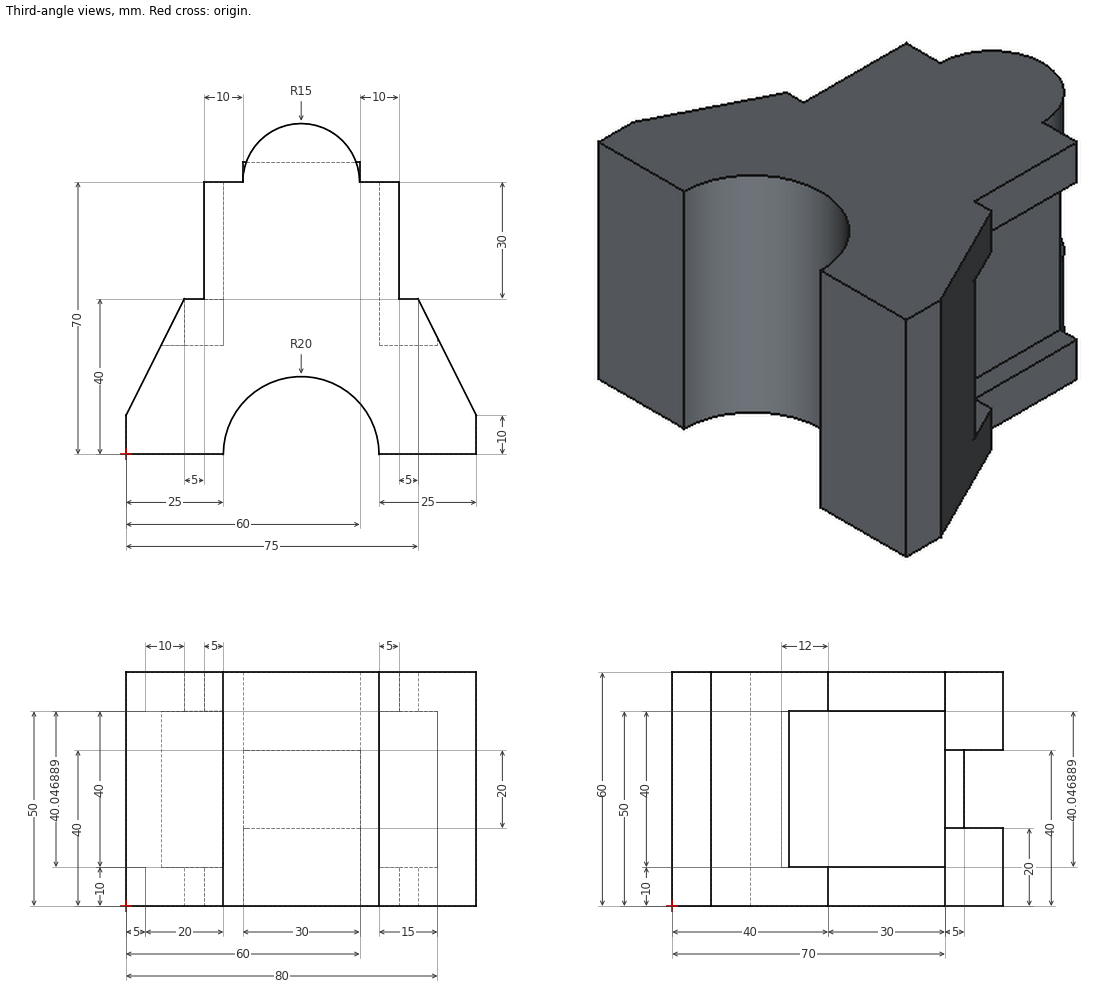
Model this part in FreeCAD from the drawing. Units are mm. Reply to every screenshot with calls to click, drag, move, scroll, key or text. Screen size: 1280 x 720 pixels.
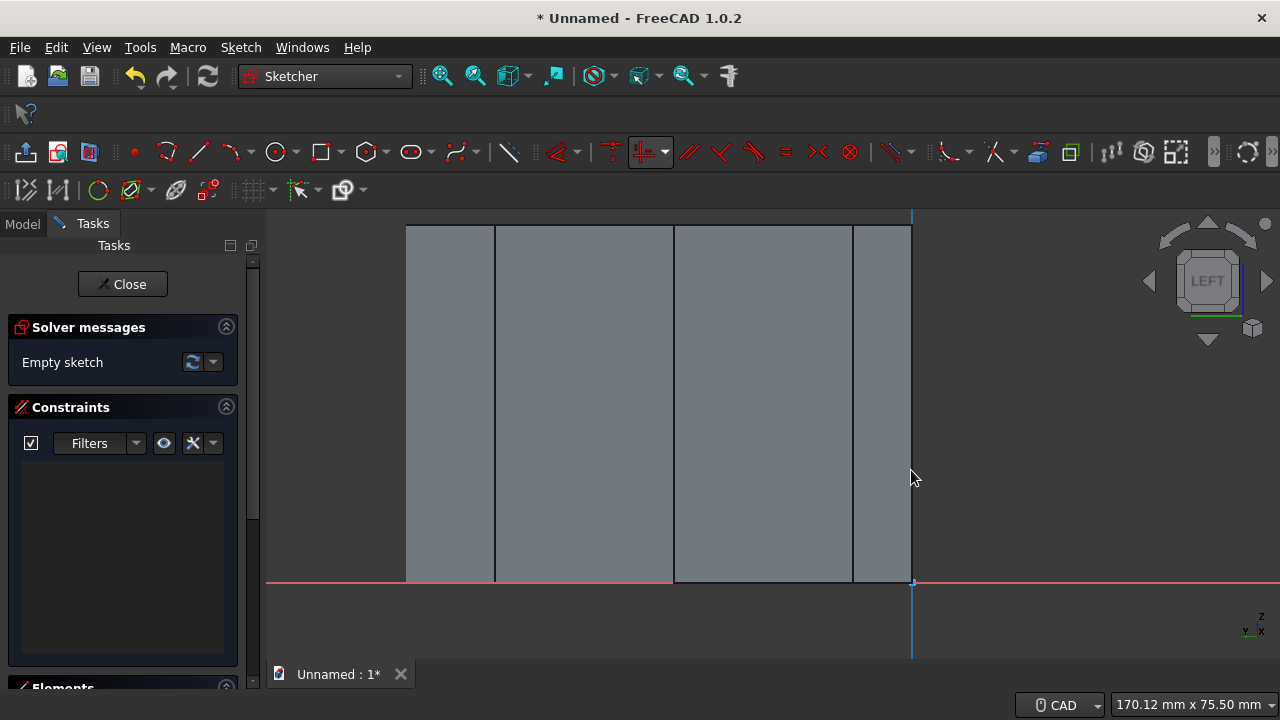
key(g)
key(r)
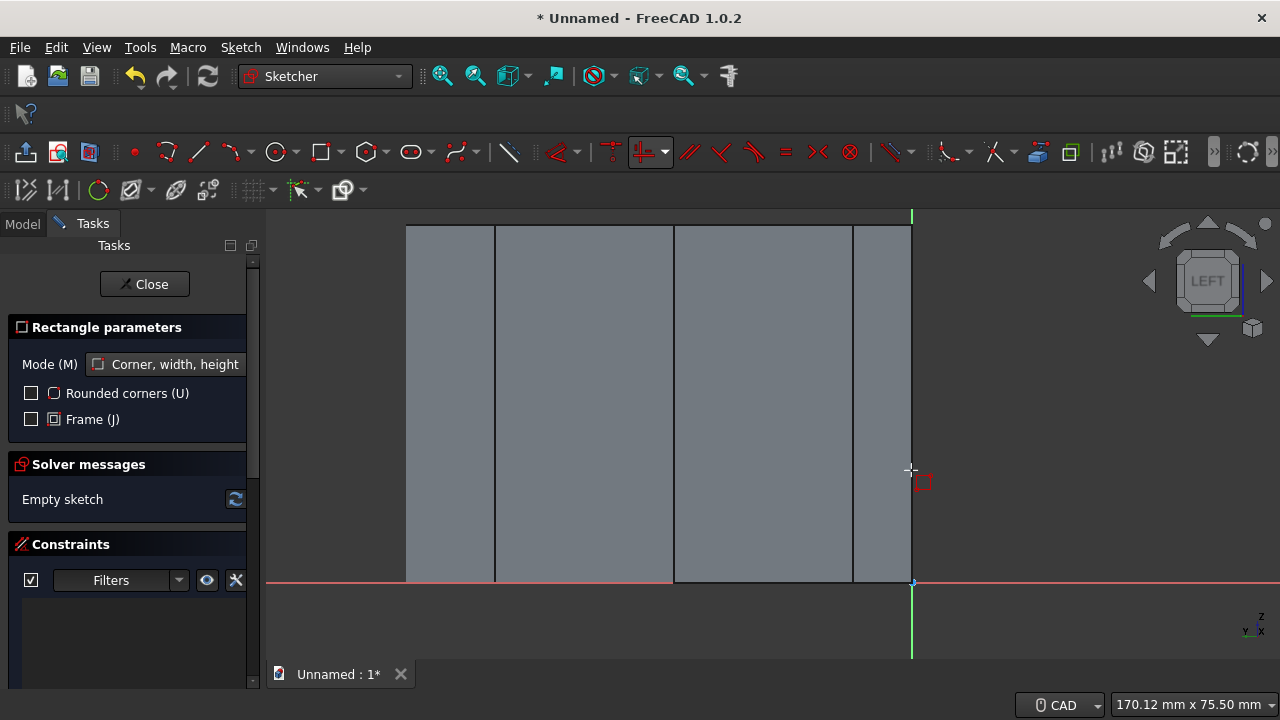
click(495, 284)
click(674, 523)
key(Escape)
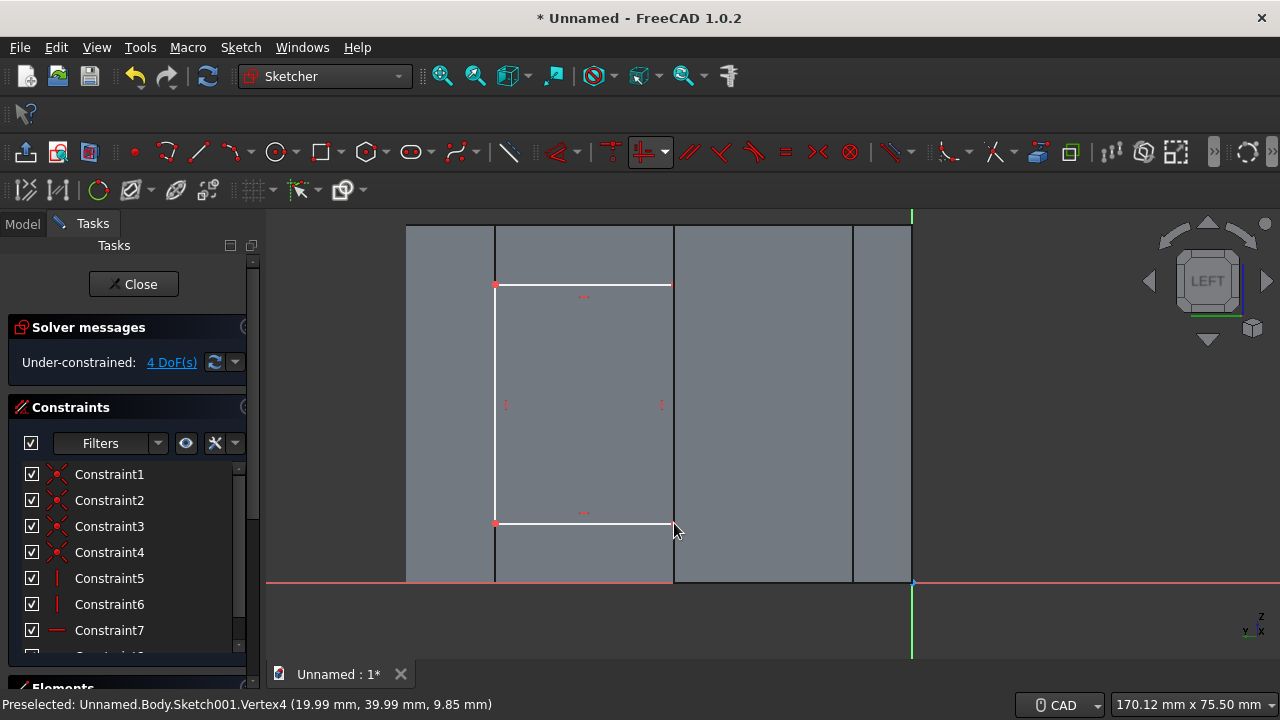
key(d)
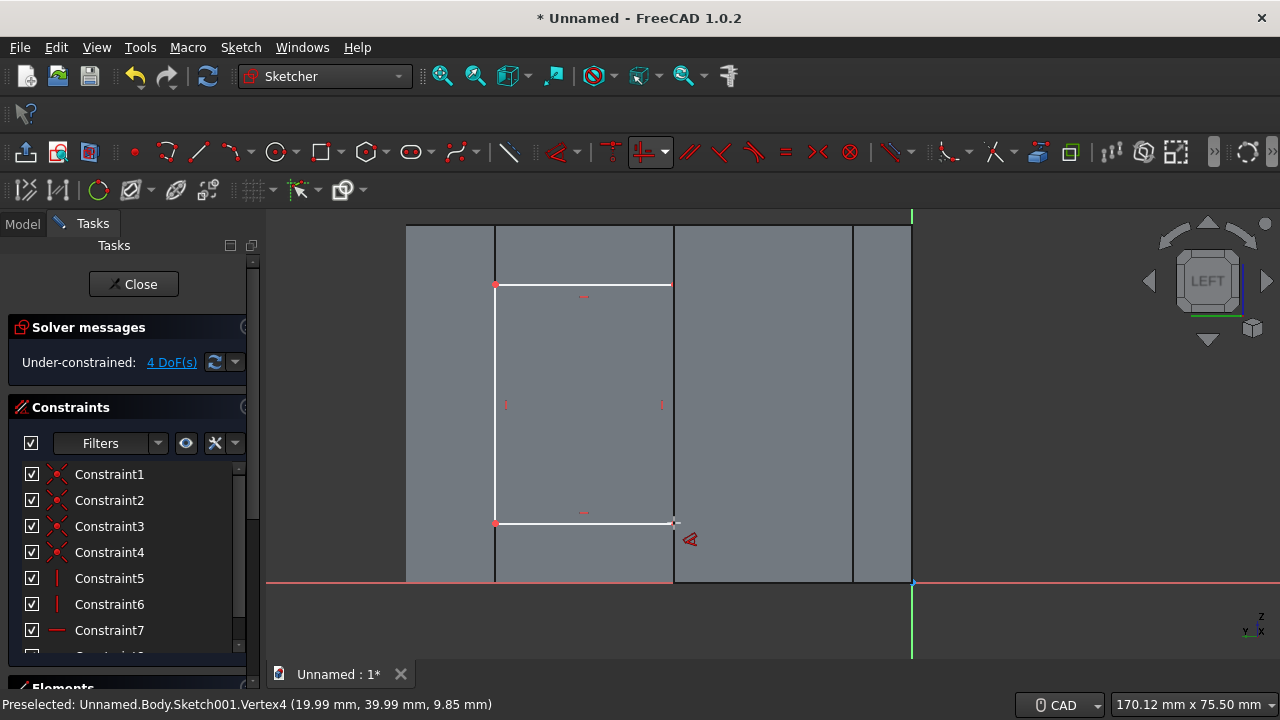
click(549, 524)
click(584, 558)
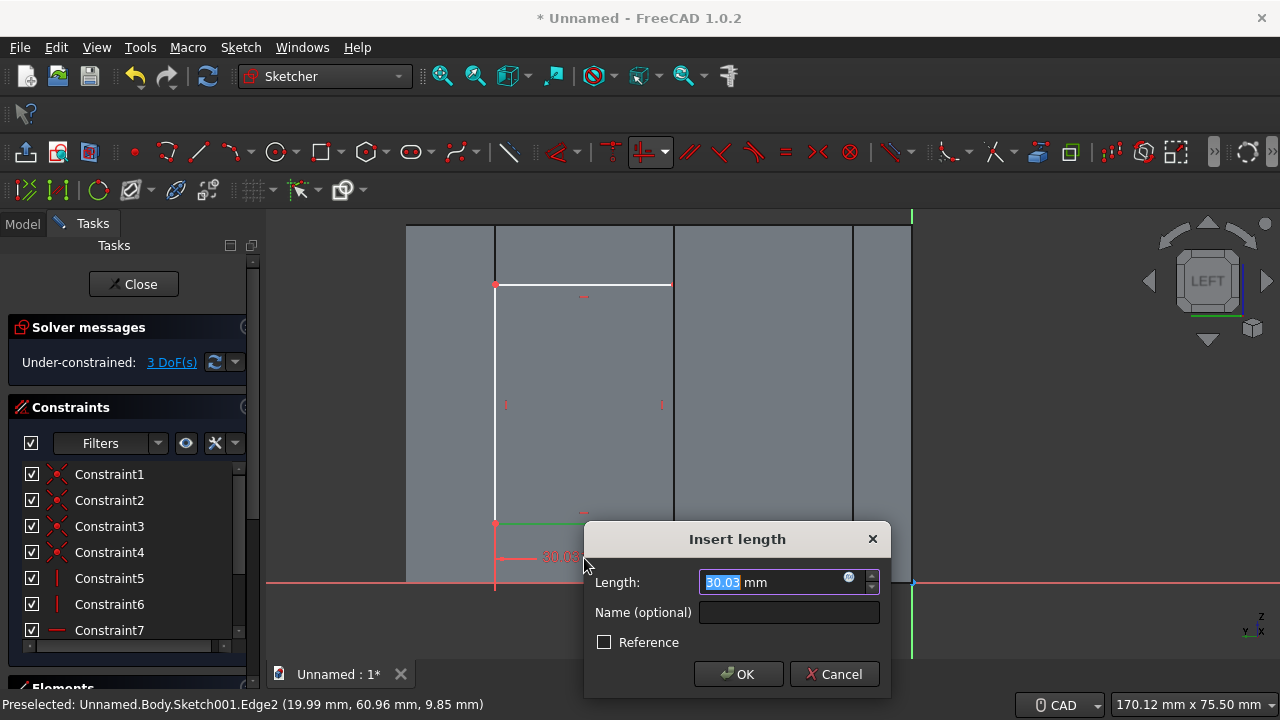
text(30)
key(Return)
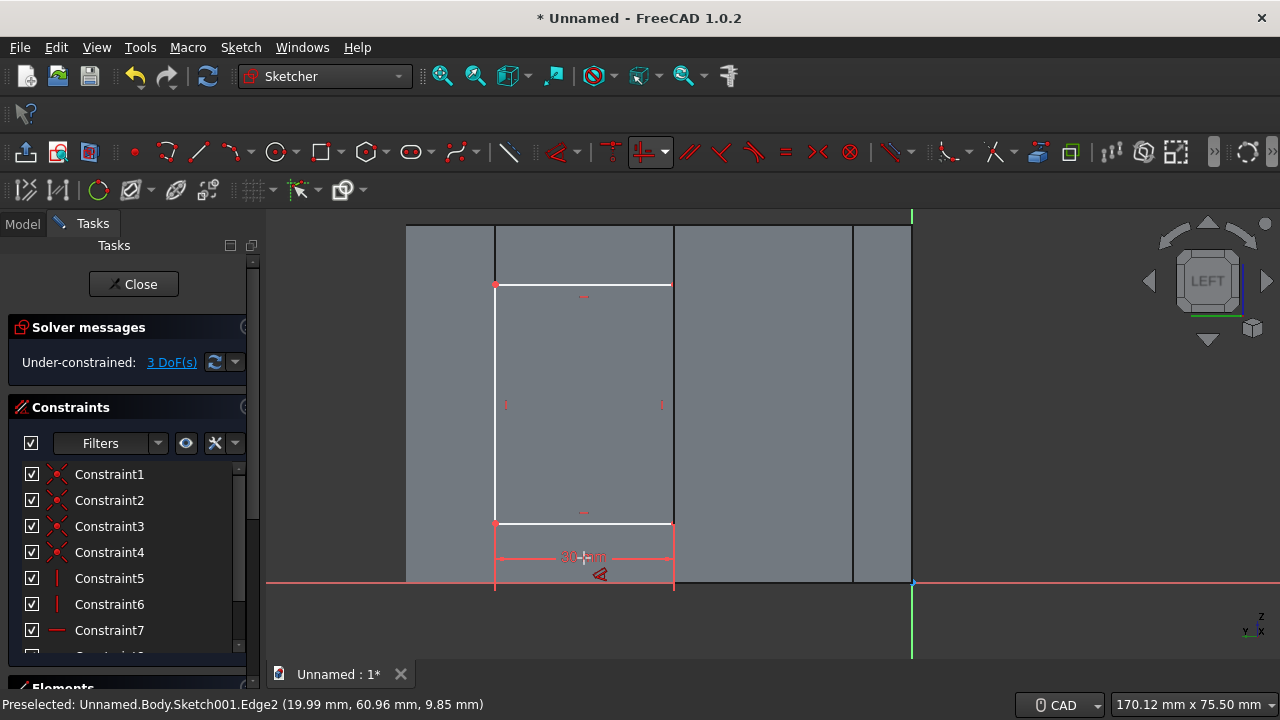
click(495, 285)
click(704, 617)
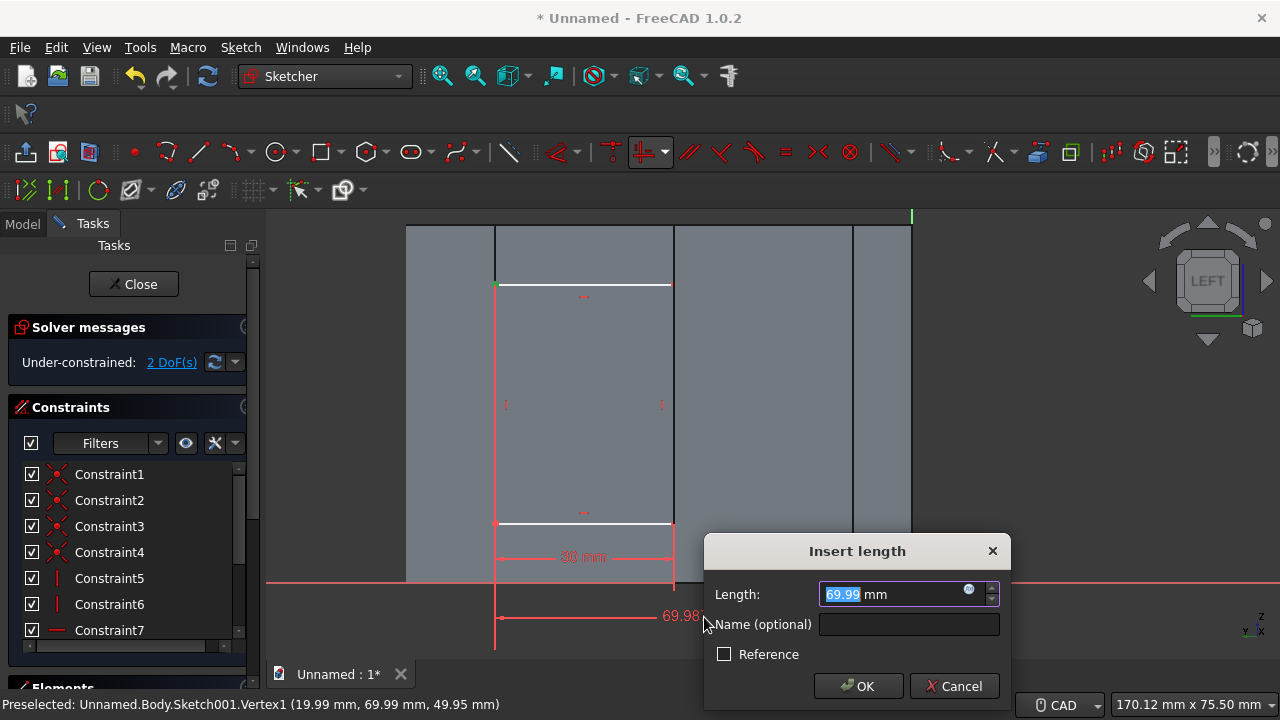
text(70)
key(Return)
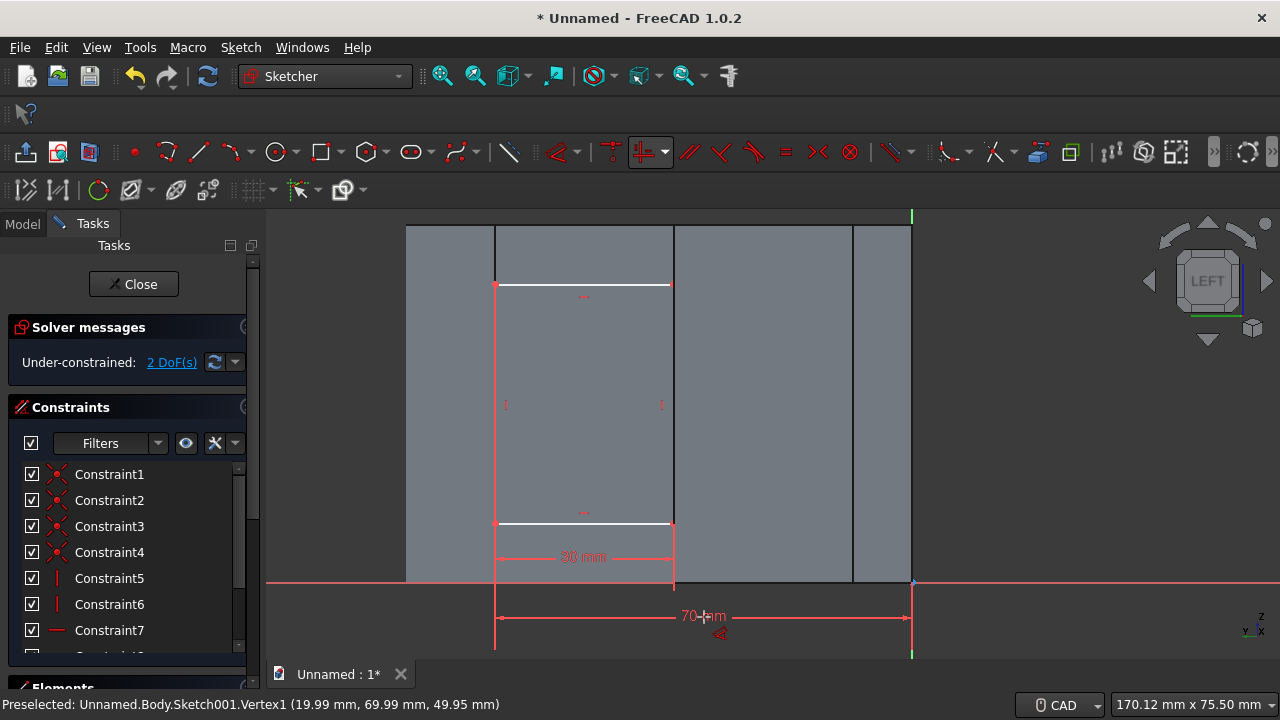
click(495, 524)
click(946, 553)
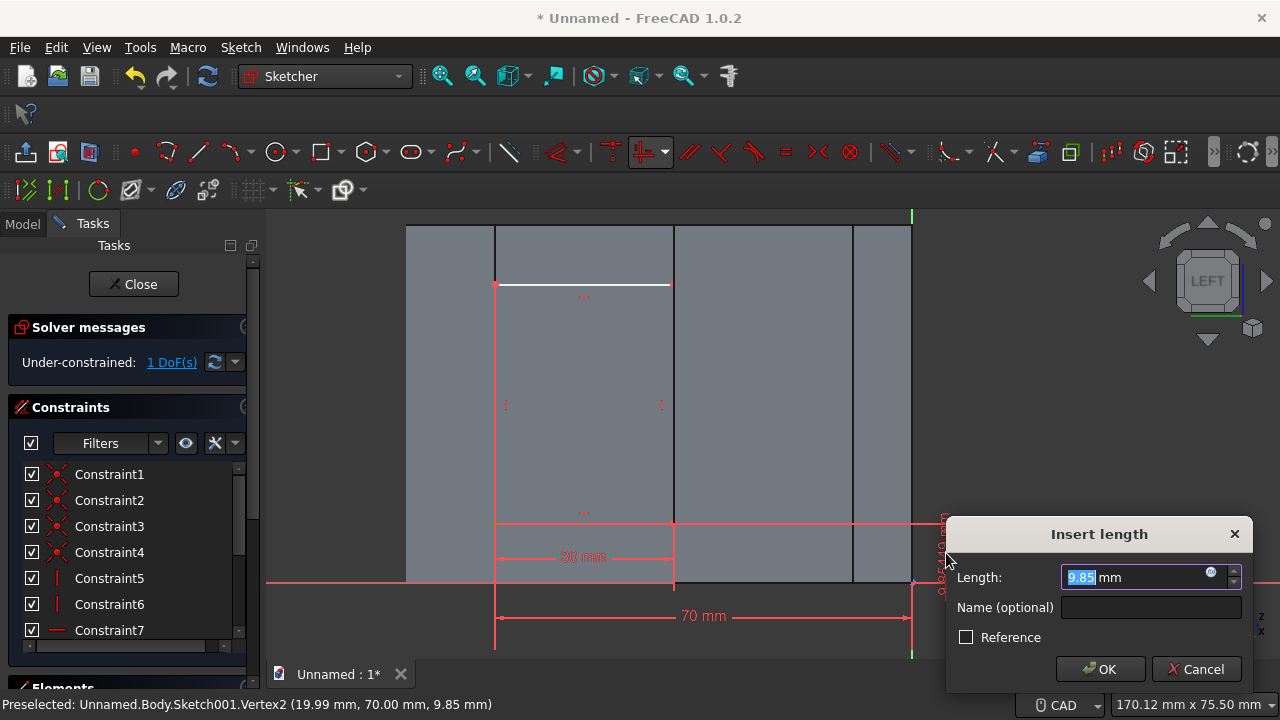
text(10)
key(Return)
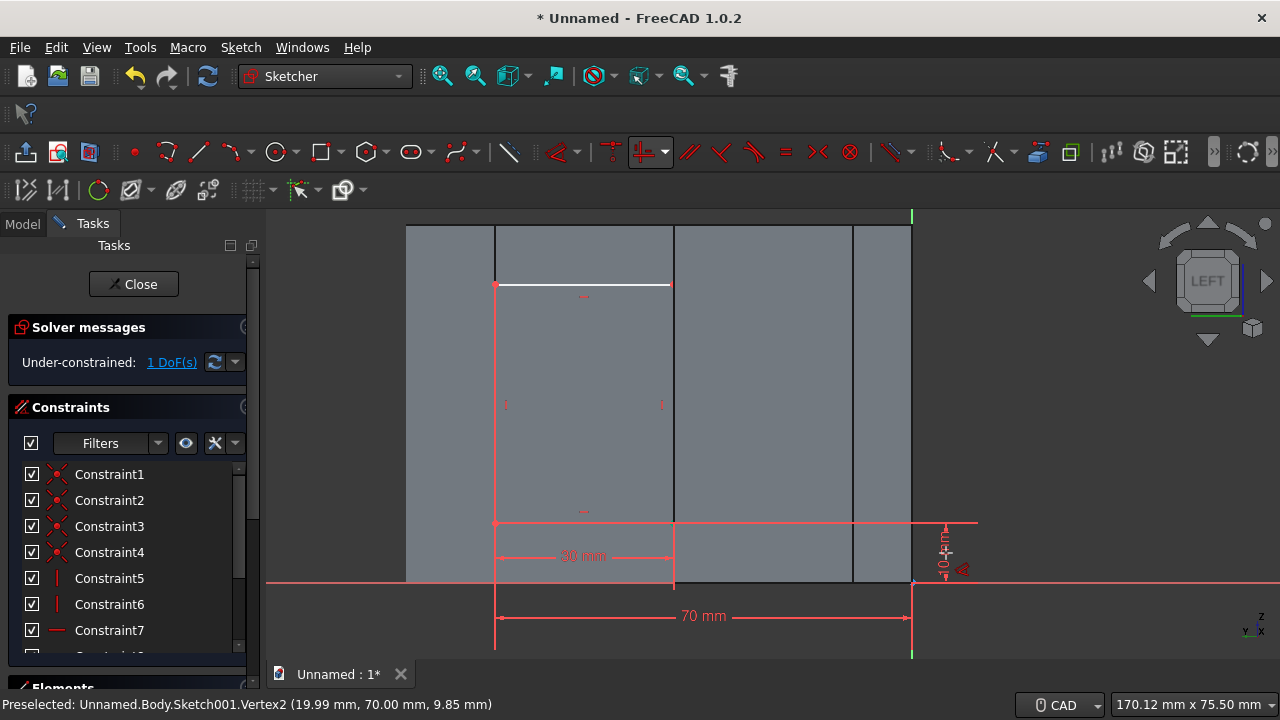
click(495, 356)
click(461, 404)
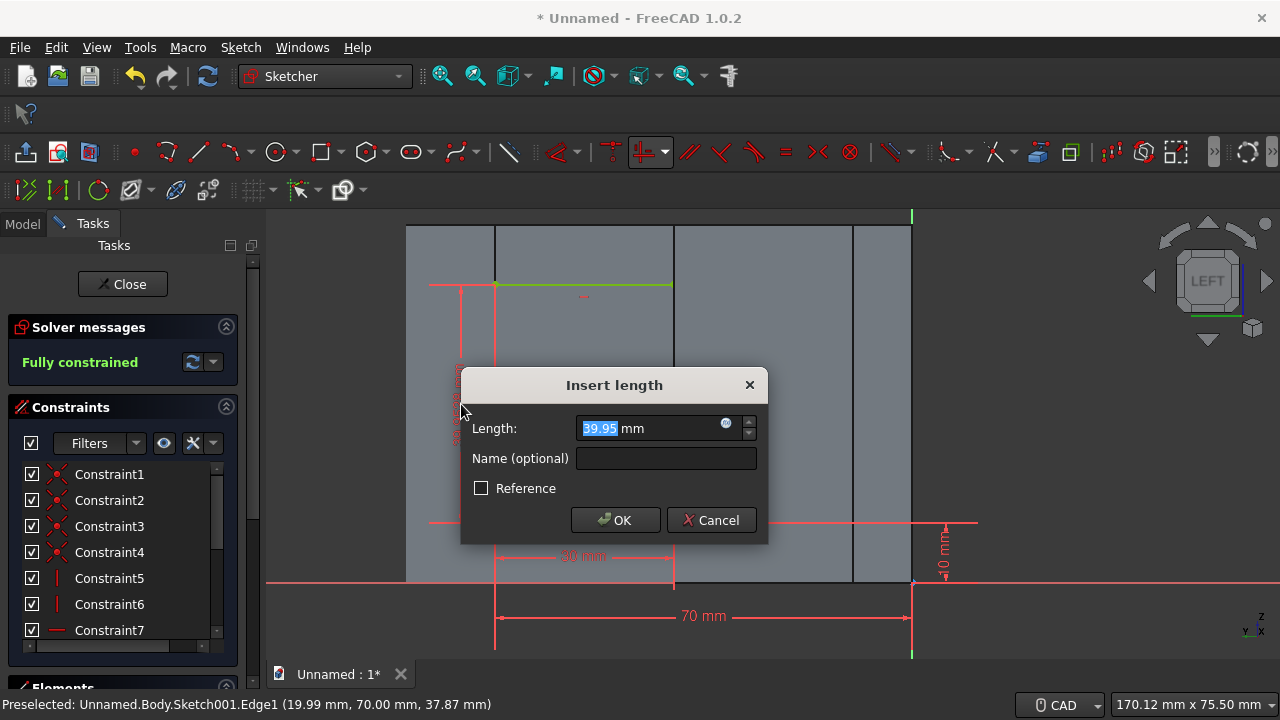
text(40.046889)
key(Return)
key(Escape)